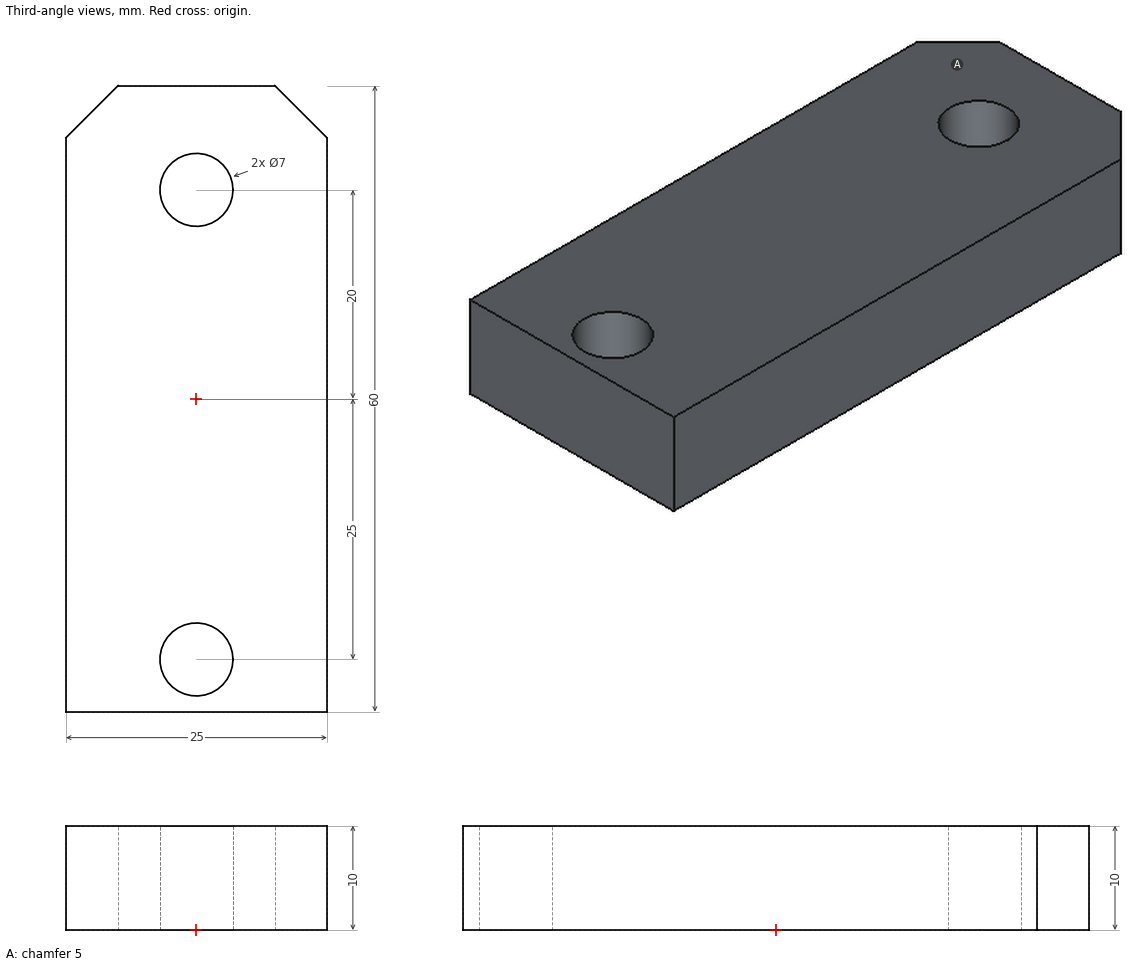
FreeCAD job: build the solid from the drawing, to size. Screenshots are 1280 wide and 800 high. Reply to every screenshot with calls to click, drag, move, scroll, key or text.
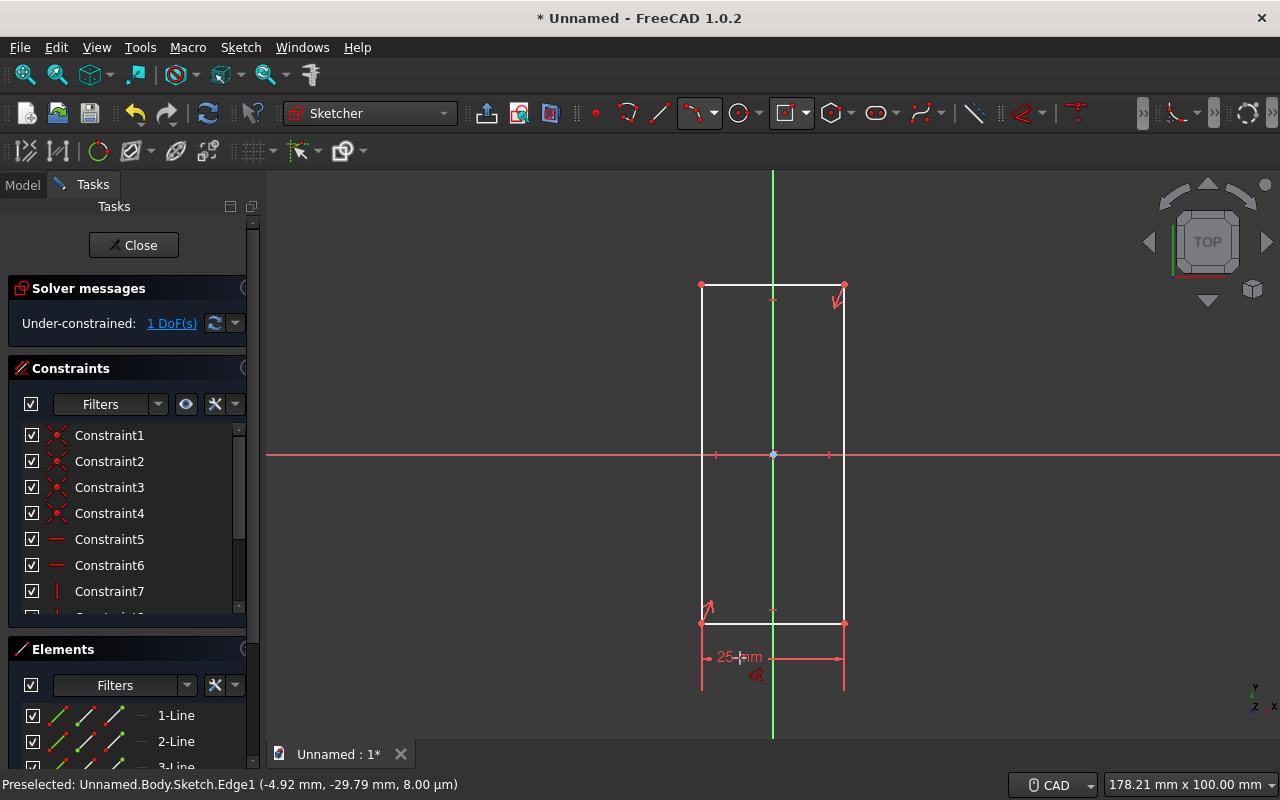
click(844, 522)
click(878, 377)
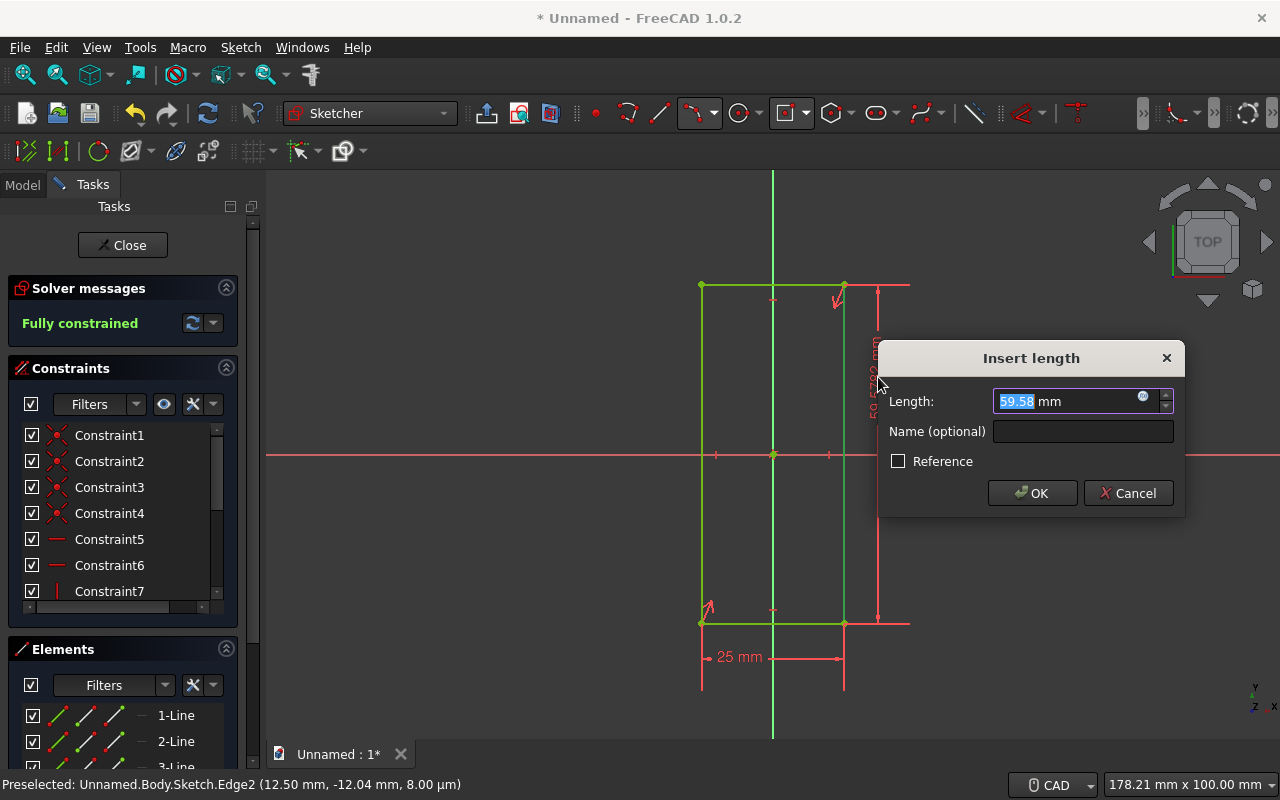
text(60)
key(Return)
key(Escape)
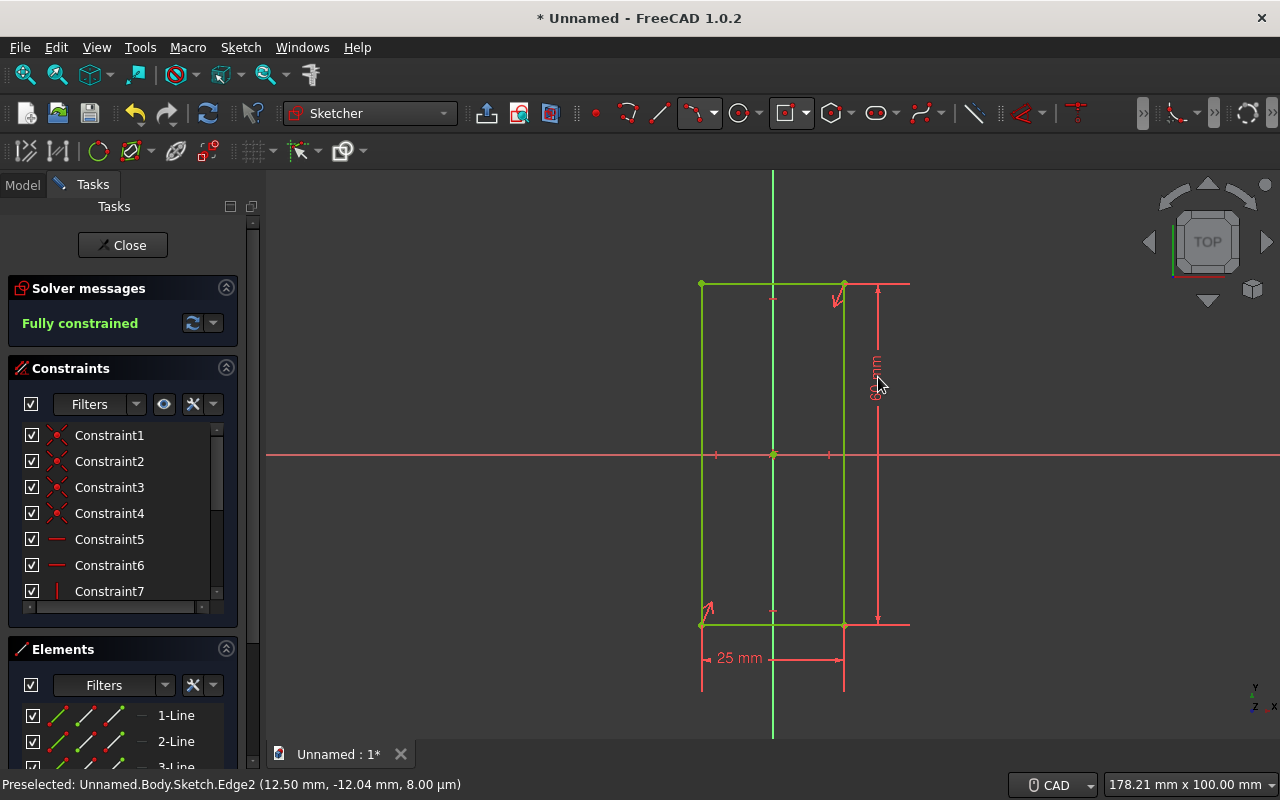
click(123, 245)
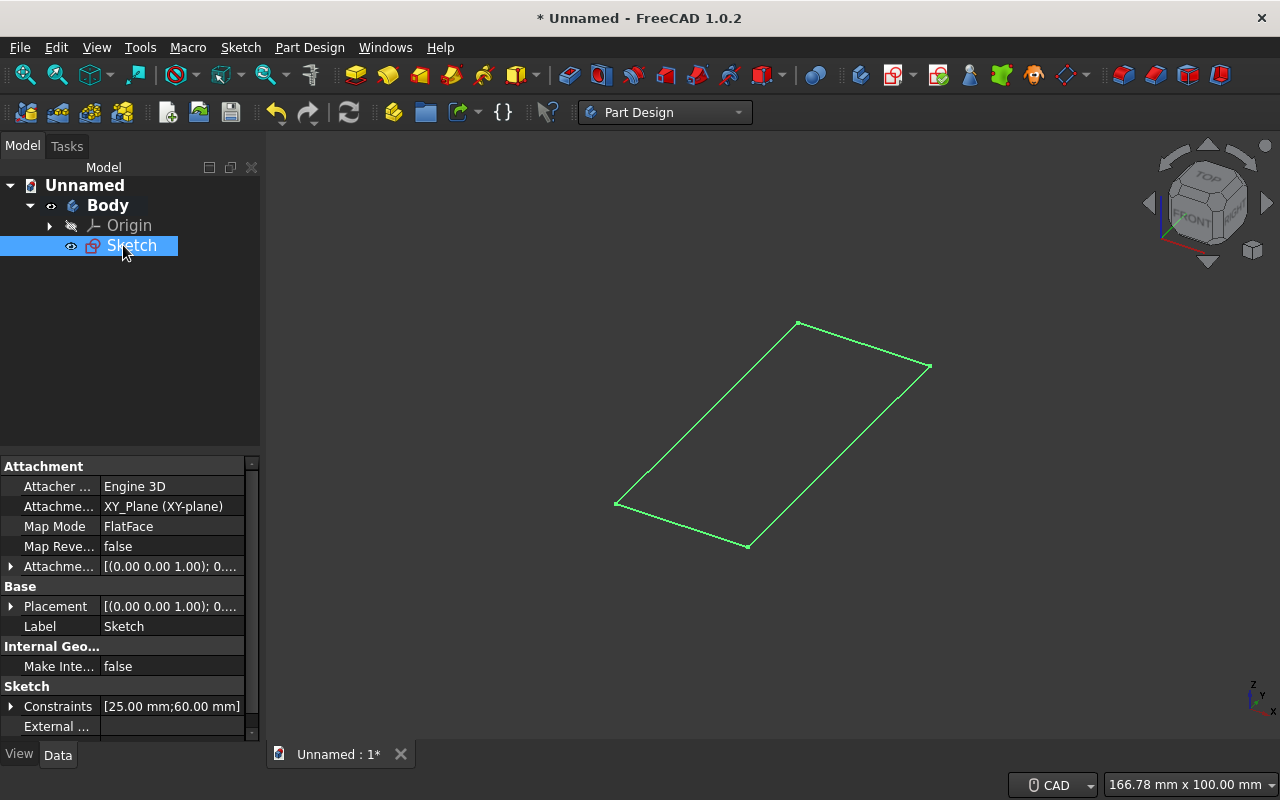
click(356, 76)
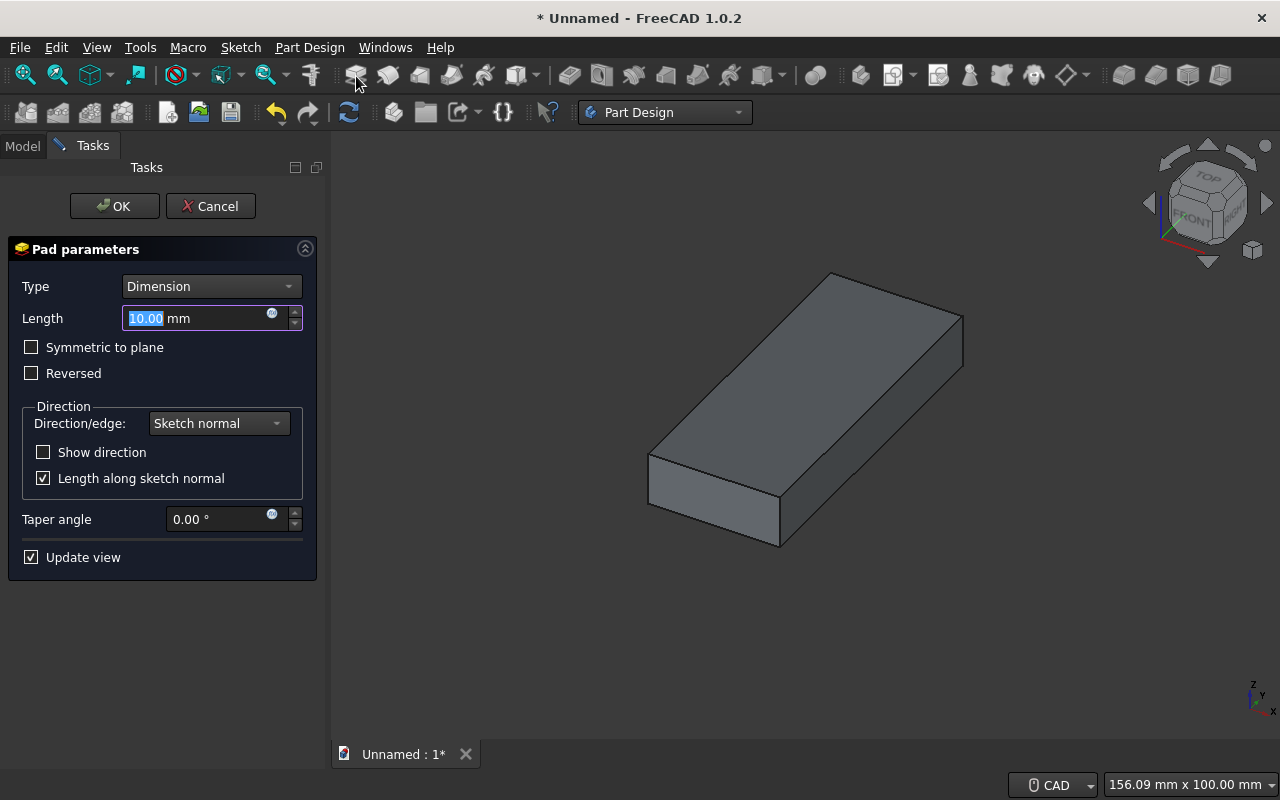
text(10)
key(Tab)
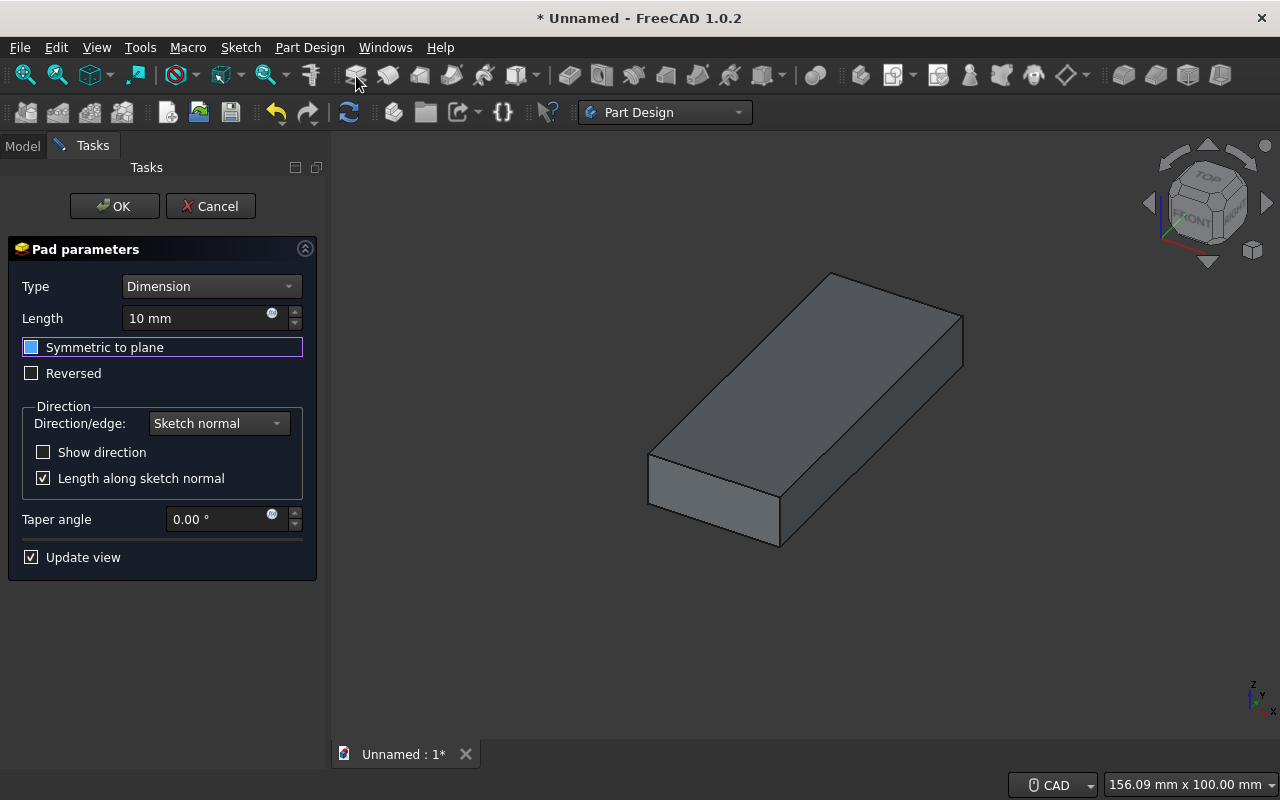
click(115, 206)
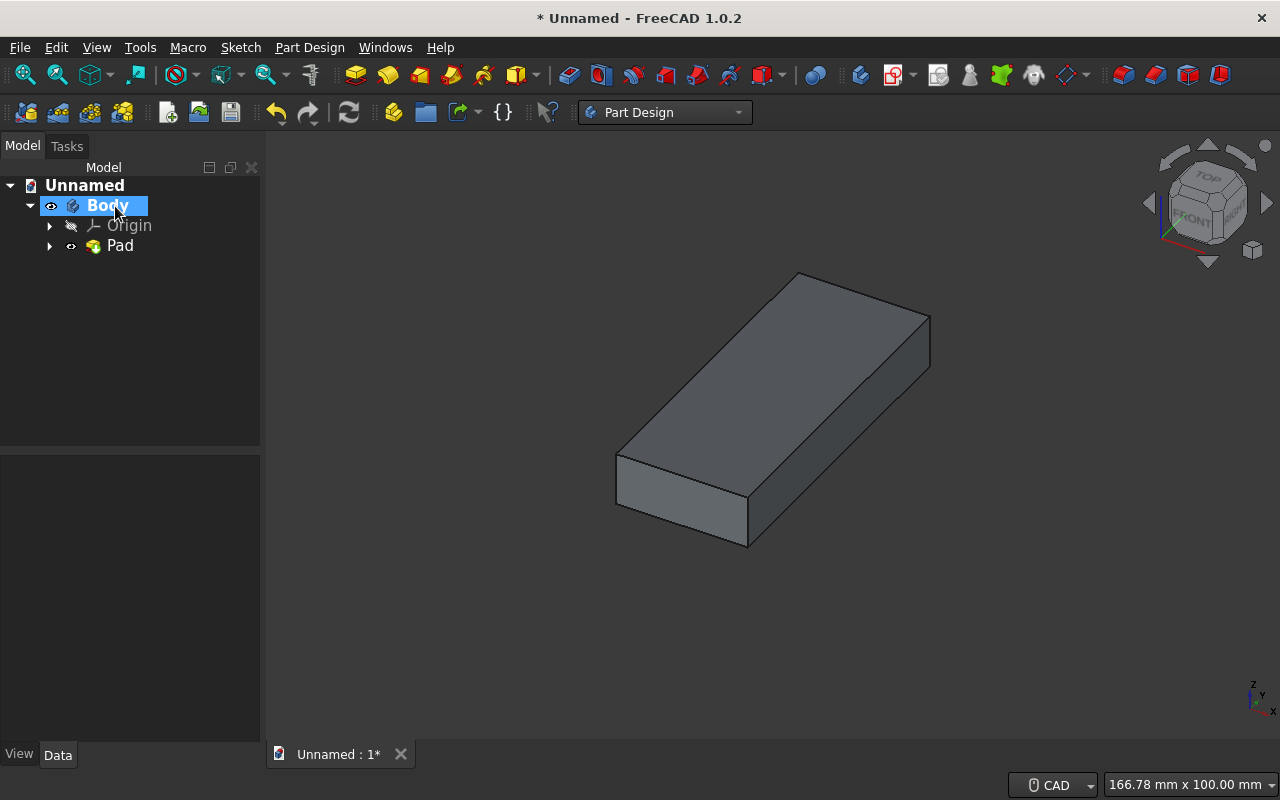
click(825, 332)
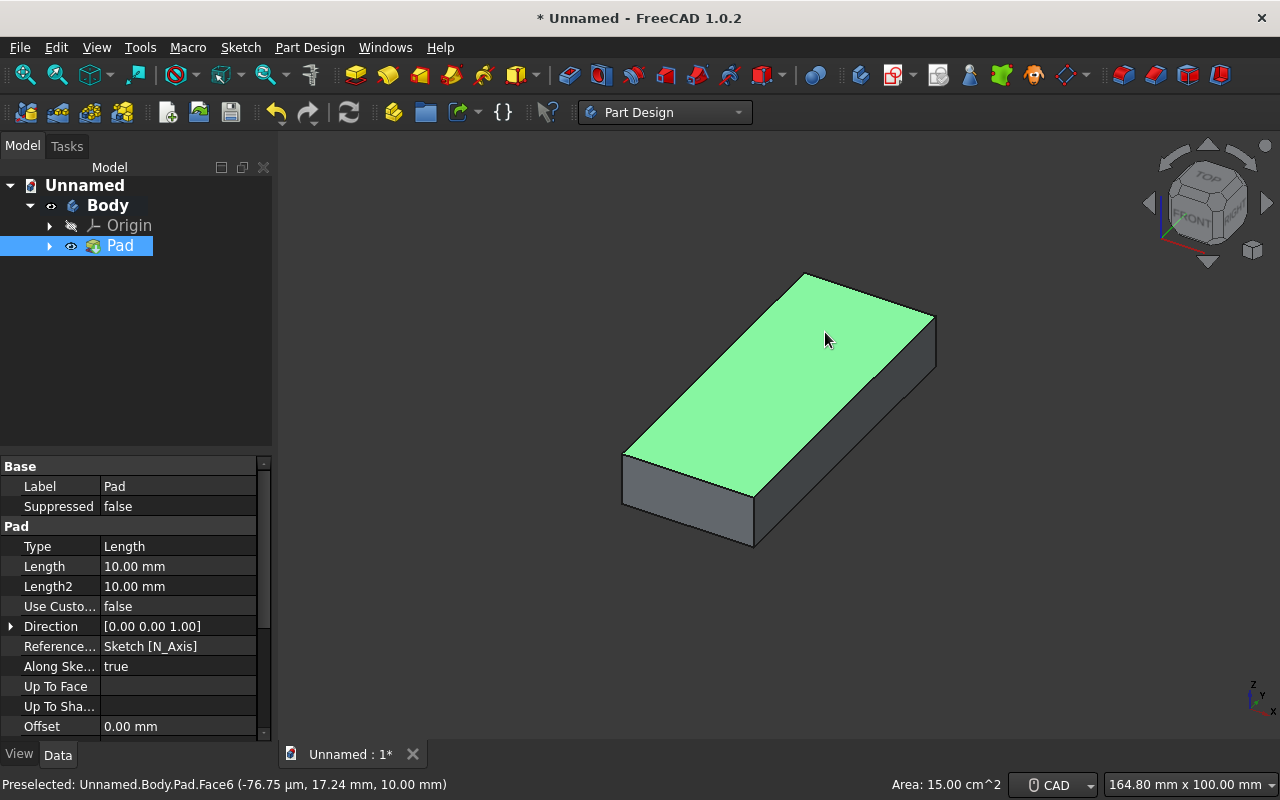
click(894, 76)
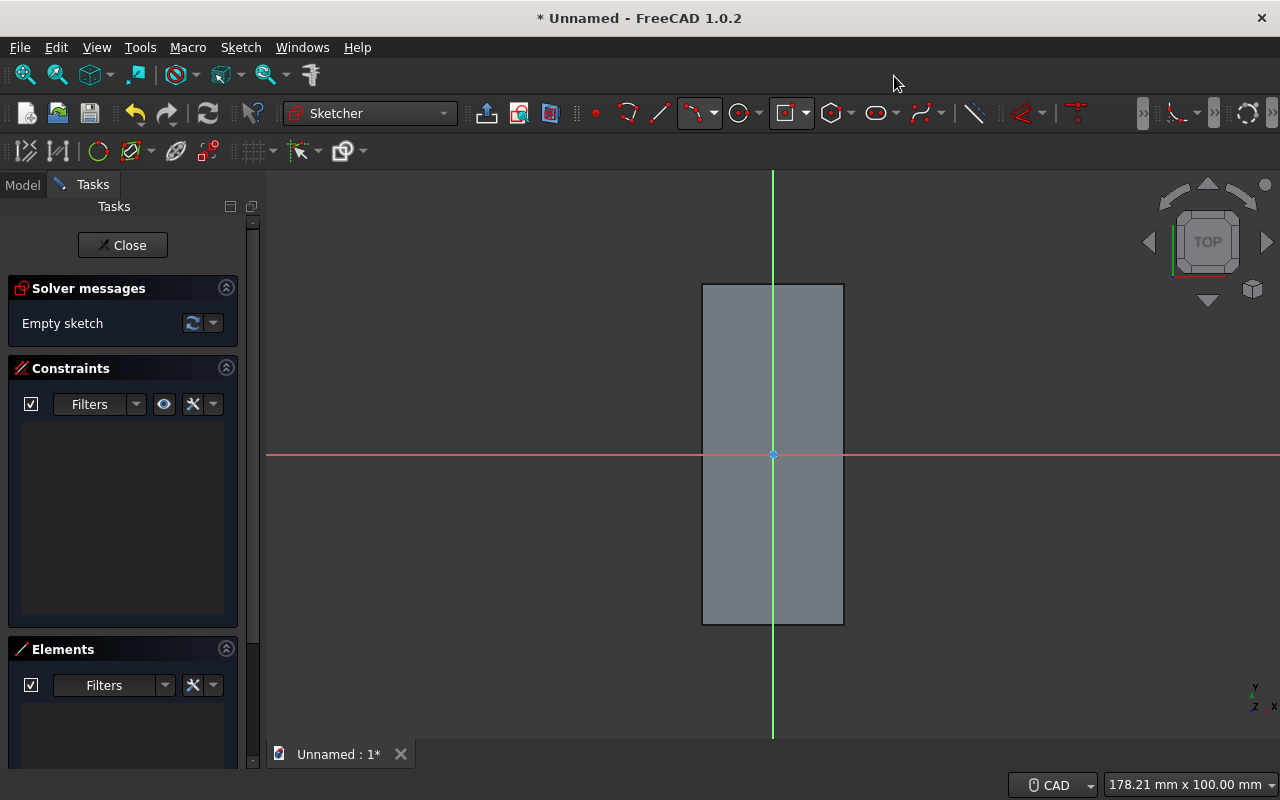
click(740, 114)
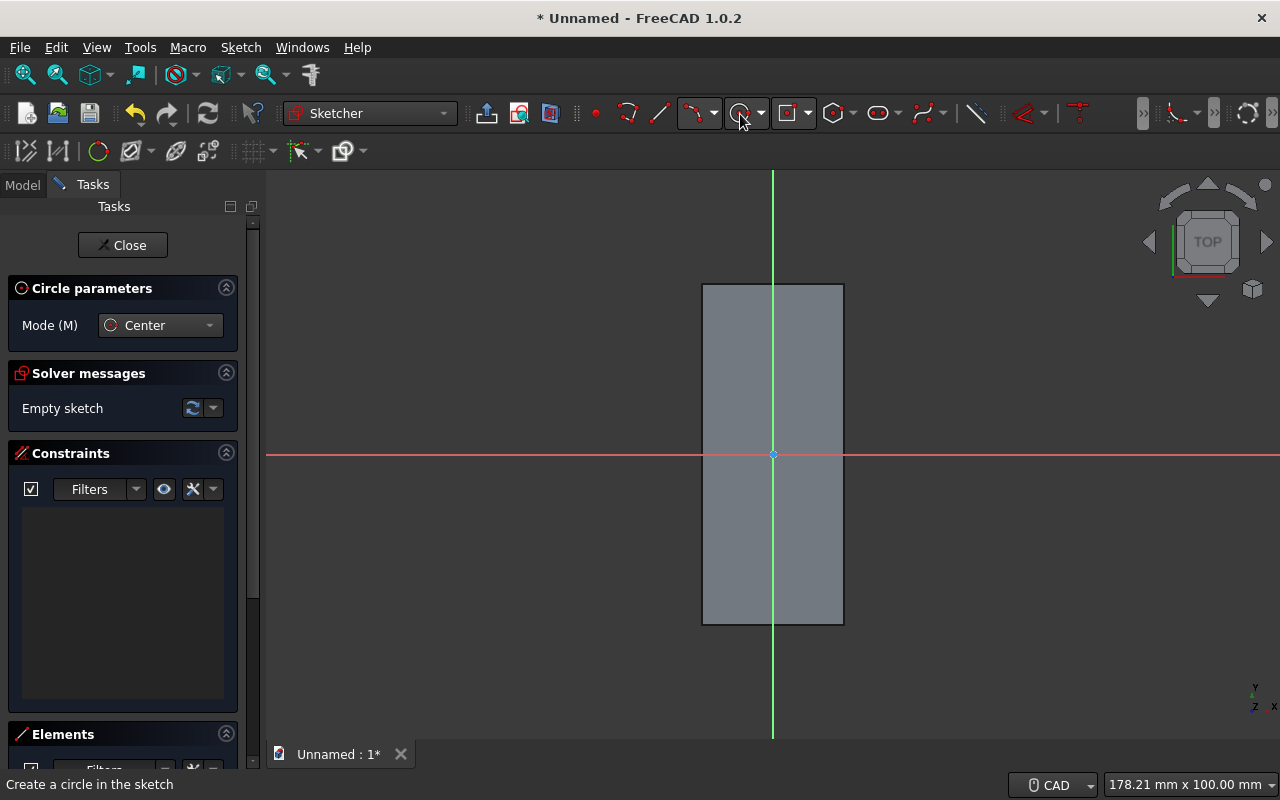
click(773, 341)
click(787, 327)